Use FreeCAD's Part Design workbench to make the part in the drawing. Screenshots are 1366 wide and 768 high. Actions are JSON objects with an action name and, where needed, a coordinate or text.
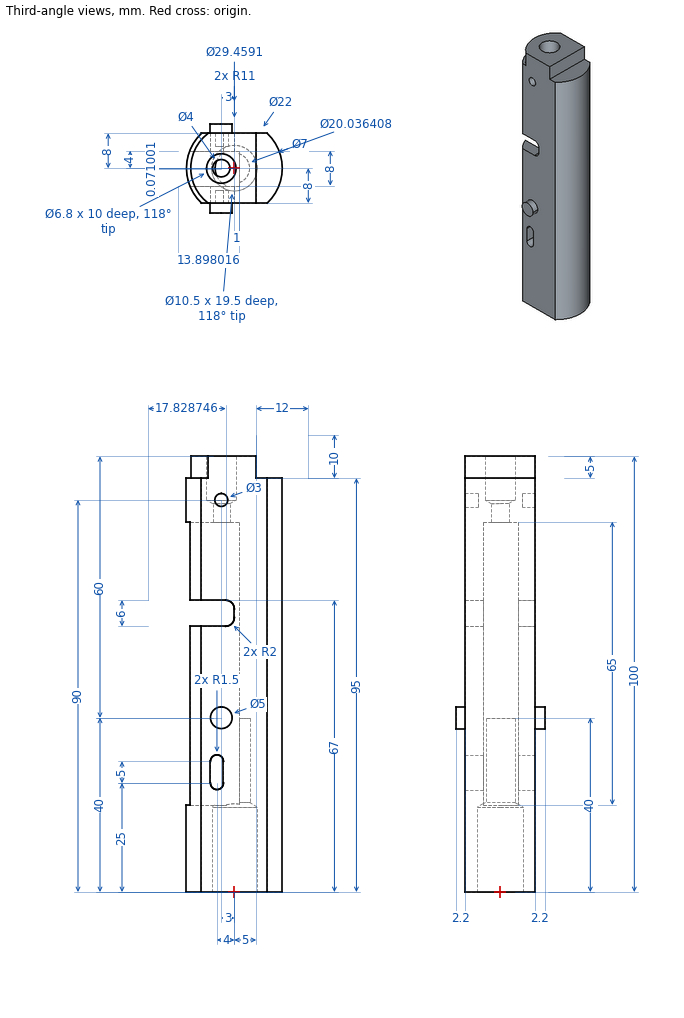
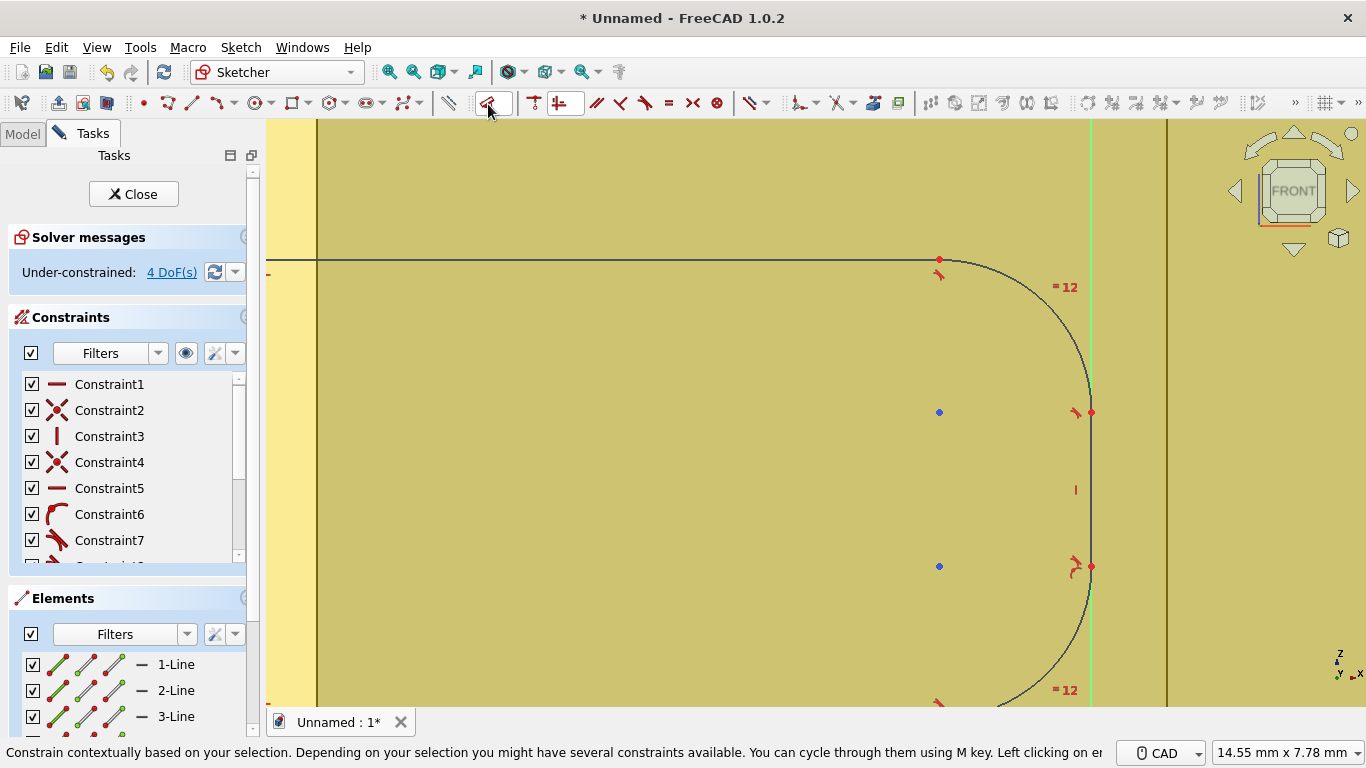
{"action": "left_click", "coordinate": [1075, 635]}
{"action": "left_click", "coordinate": [1123, 561]}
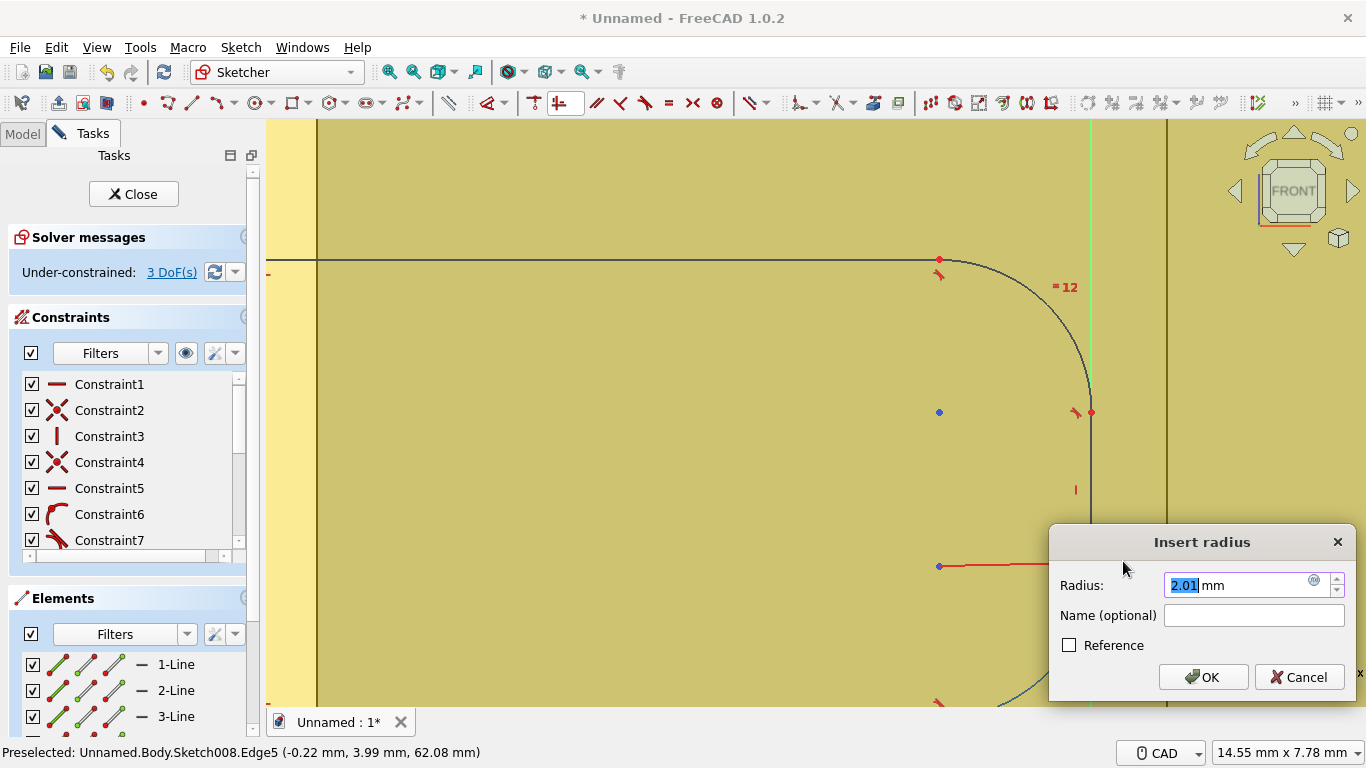
{"action": "type", "text": "2"}
{"action": "key", "text": "Return"}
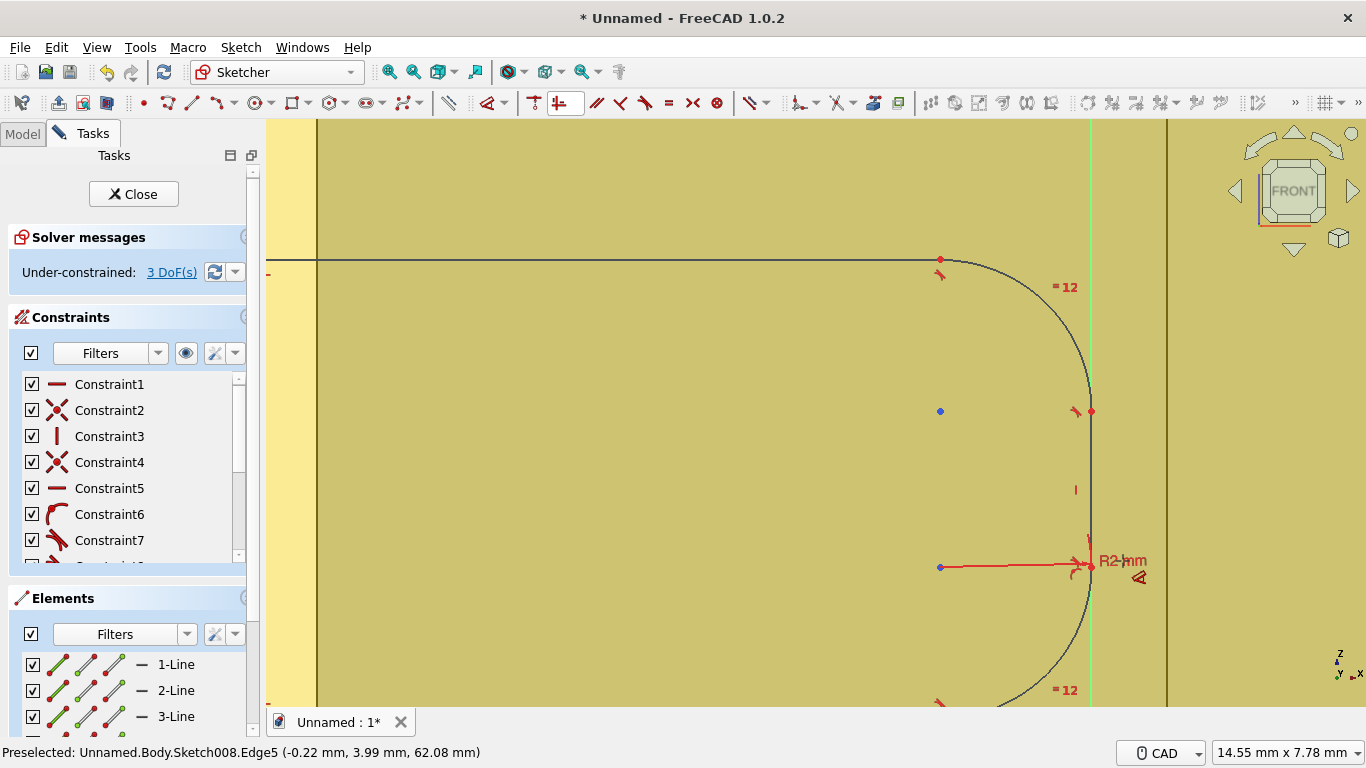
{"action": "scroll", "coordinate": [1078, 350], "scroll_direction": "down", "scroll_amount": 4}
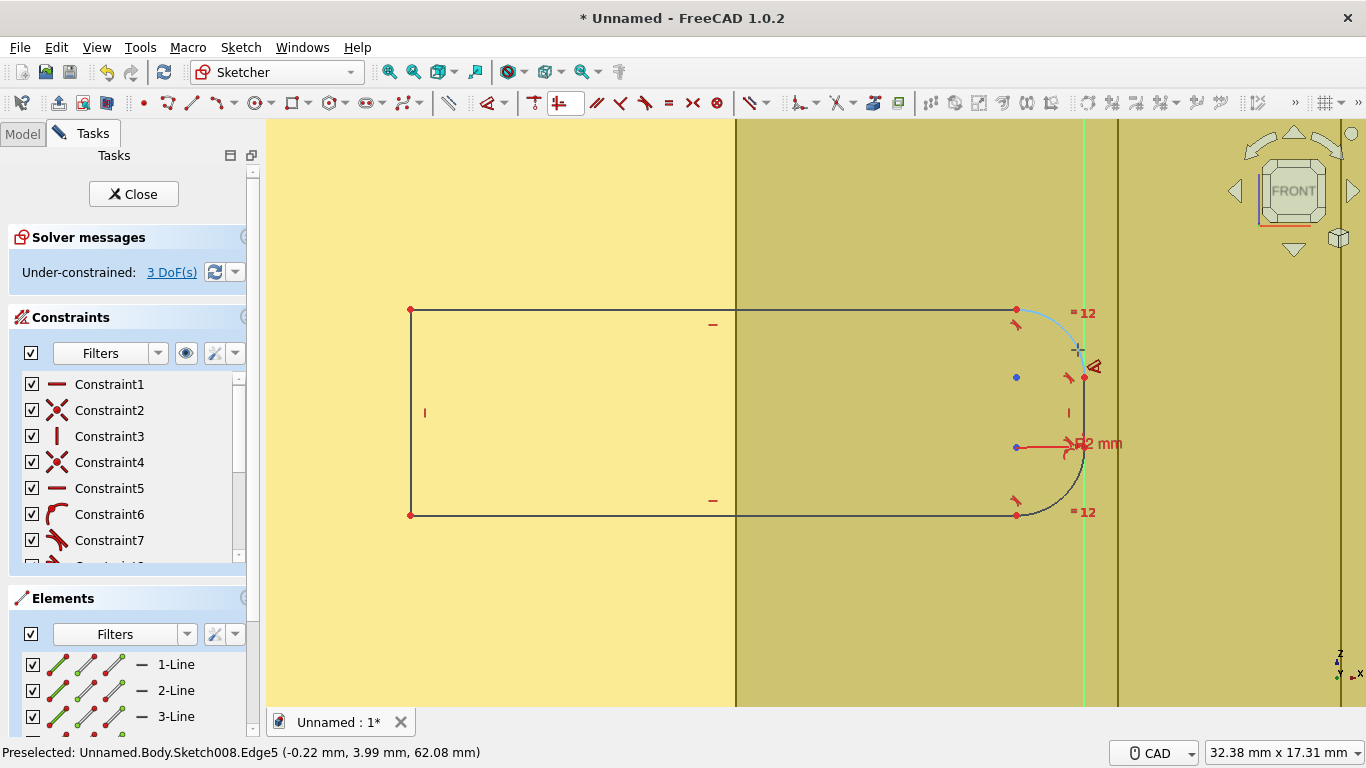
{"action": "left_click", "coordinate": [411, 372]}
{"action": "left_click", "coordinate": [377, 413]}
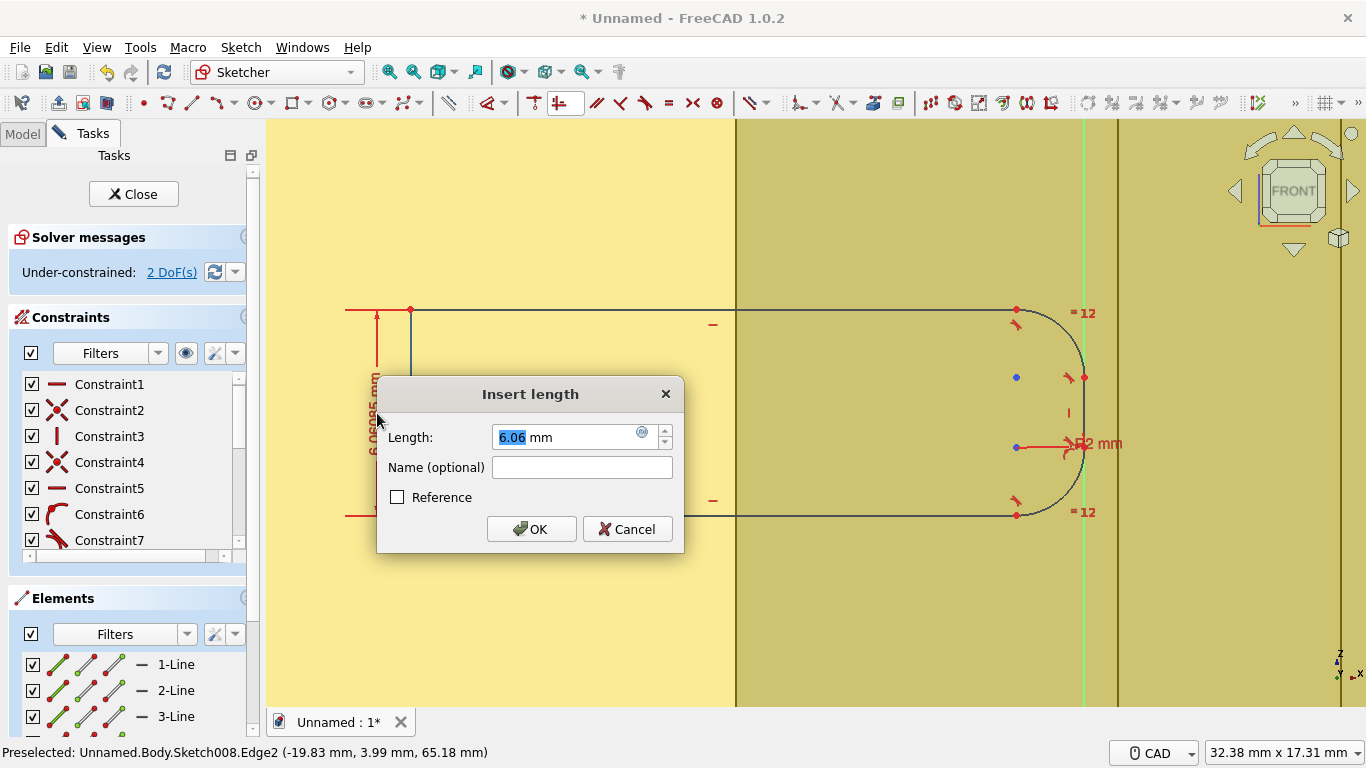
{"action": "type", "text": "6"}
{"action": "key", "text": "Return"}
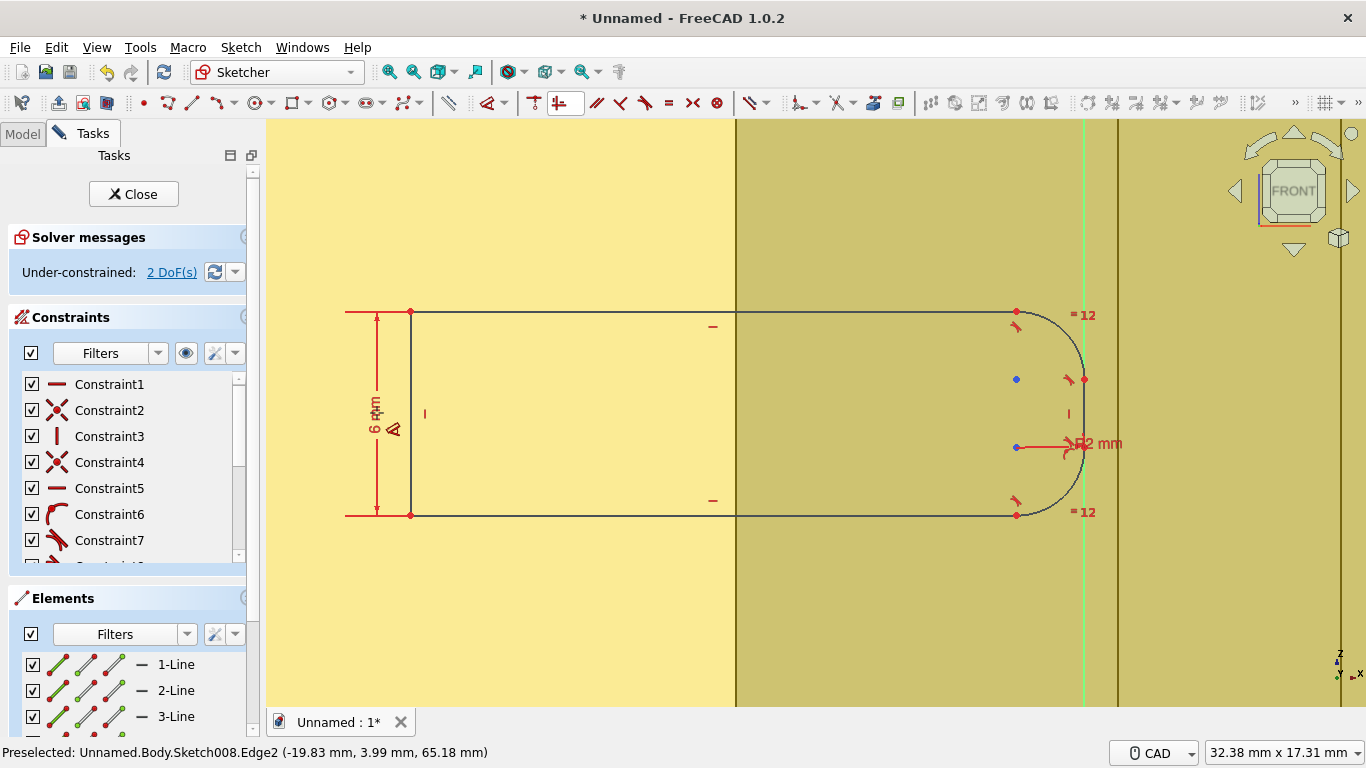
{"action": "left_click", "coordinate": [1017, 312]}
{"action": "left_click", "coordinate": [1118, 495]}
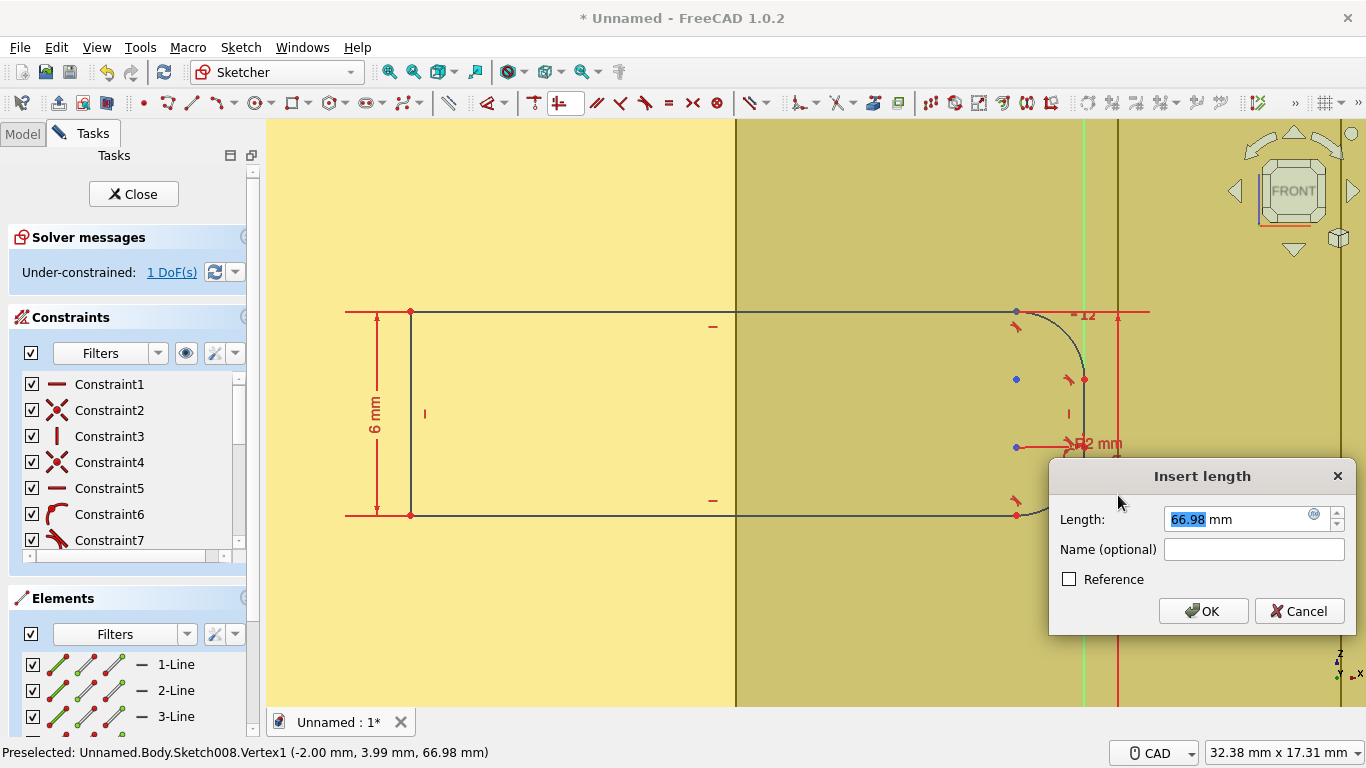
{"action": "type", "text": "67"}
{"action": "key", "text": "Return"}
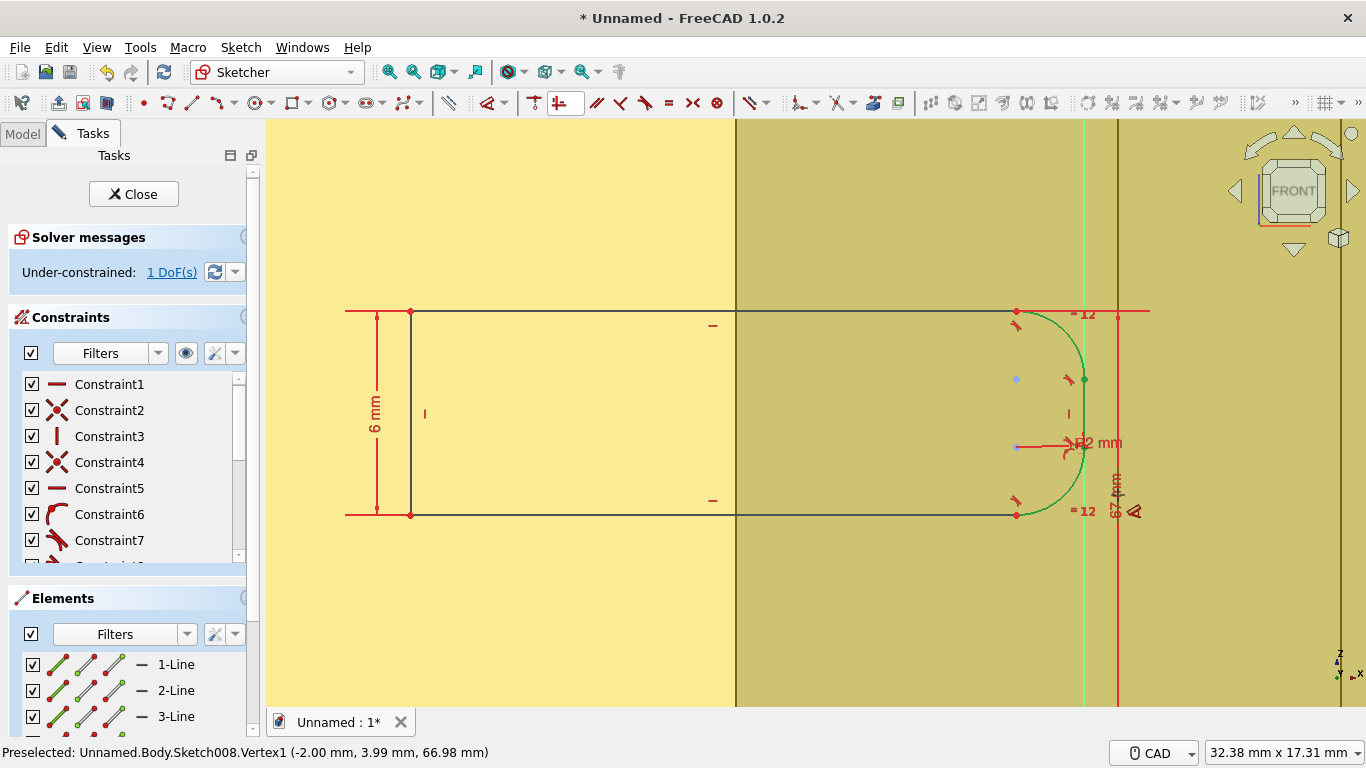
{"action": "left_click", "coordinate": [835, 311]}
{"action": "left_click", "coordinate": [714, 277]}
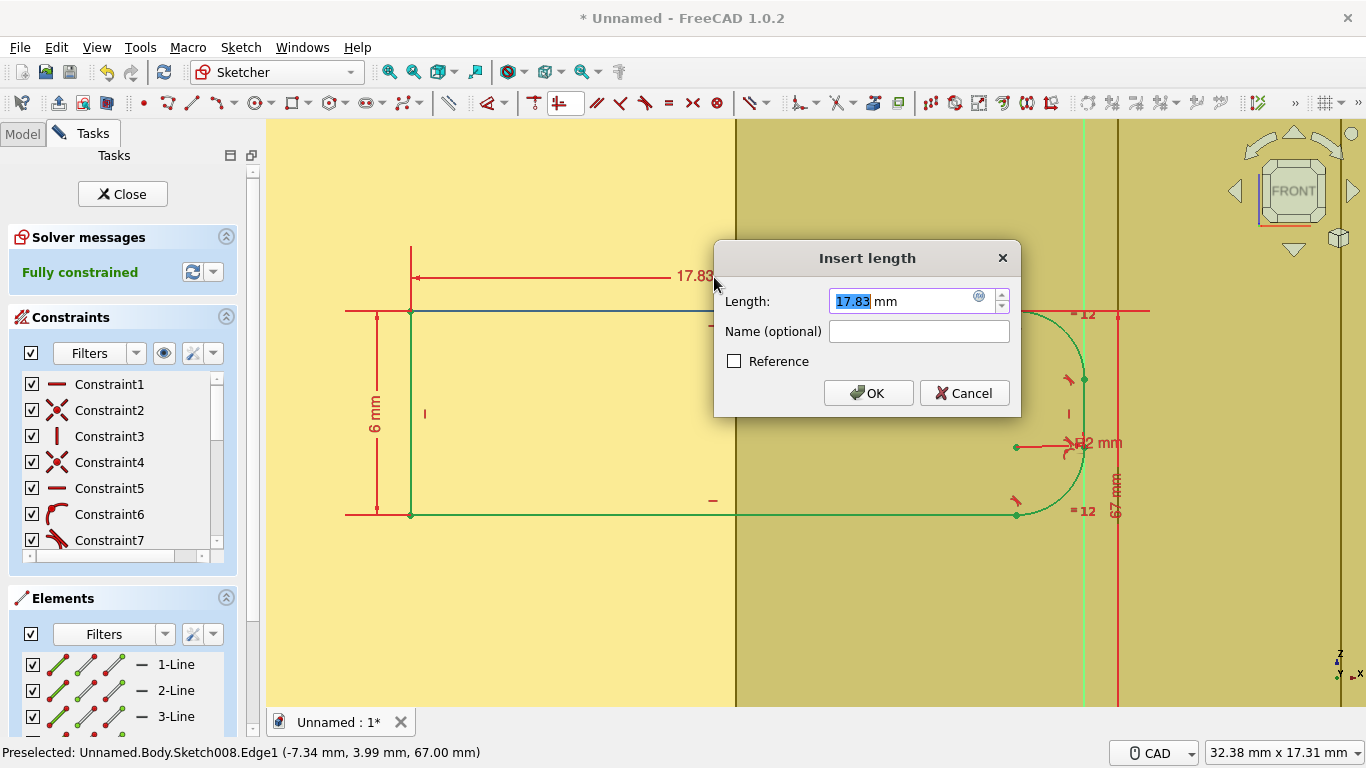
{"action": "type", "text": "17.828746"}
{"action": "key", "text": "Return"}
{"action": "key", "text": "Escape"}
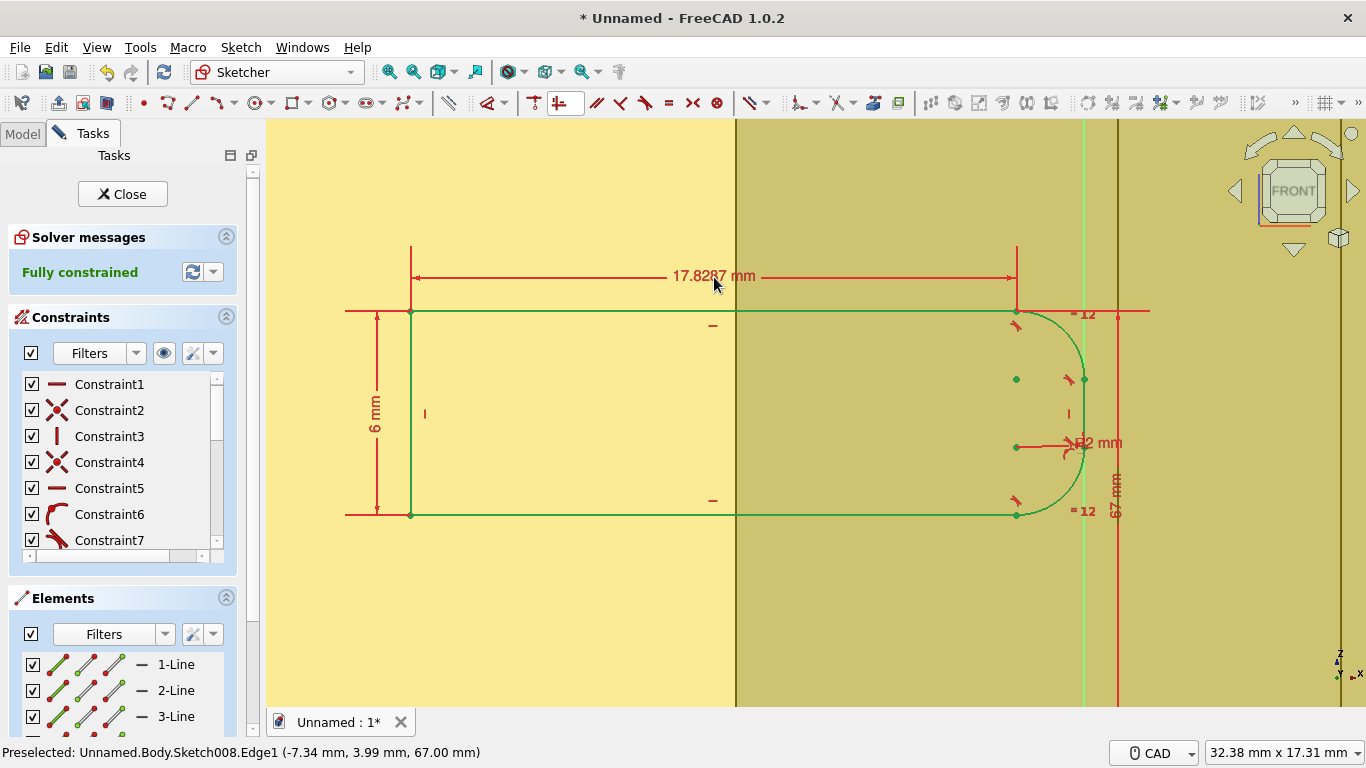
{"action": "left_click", "coordinate": [123, 194]}